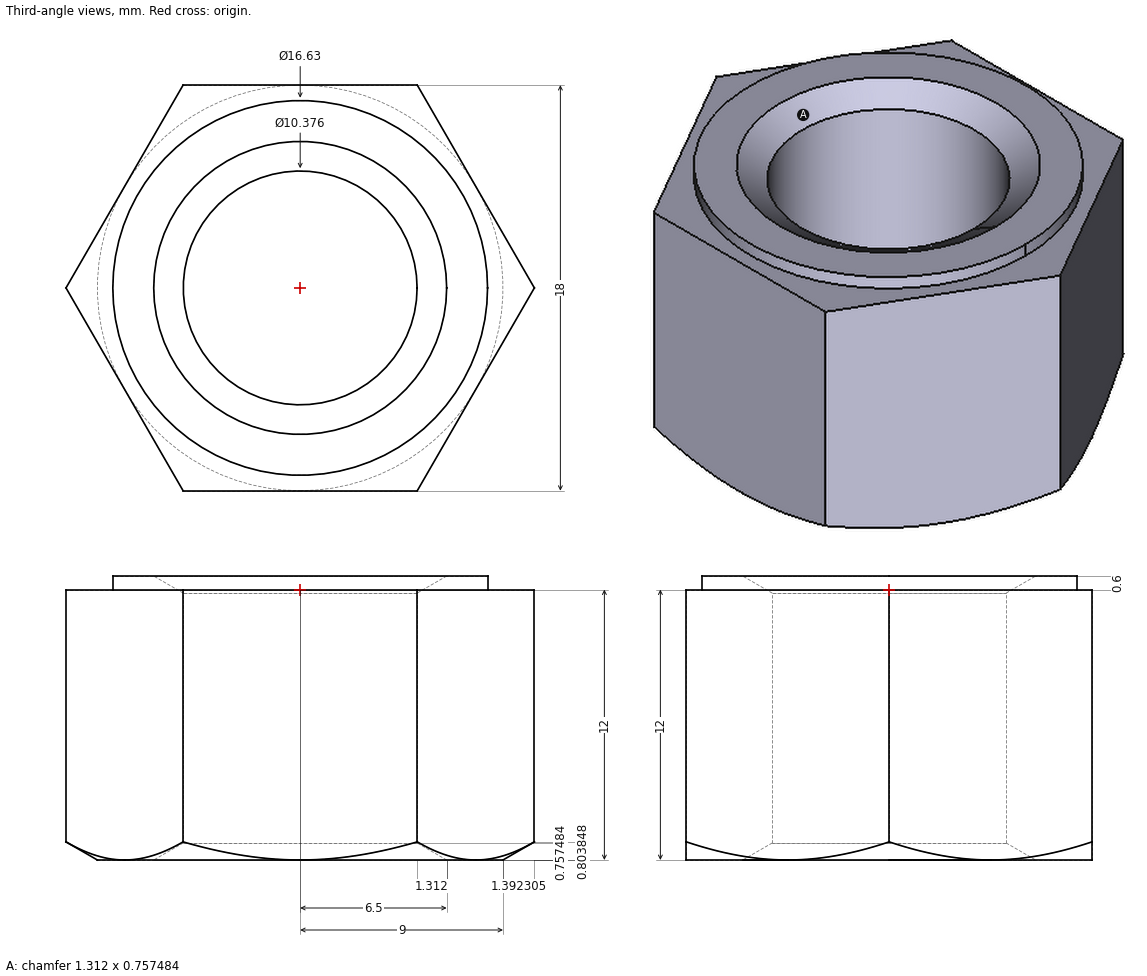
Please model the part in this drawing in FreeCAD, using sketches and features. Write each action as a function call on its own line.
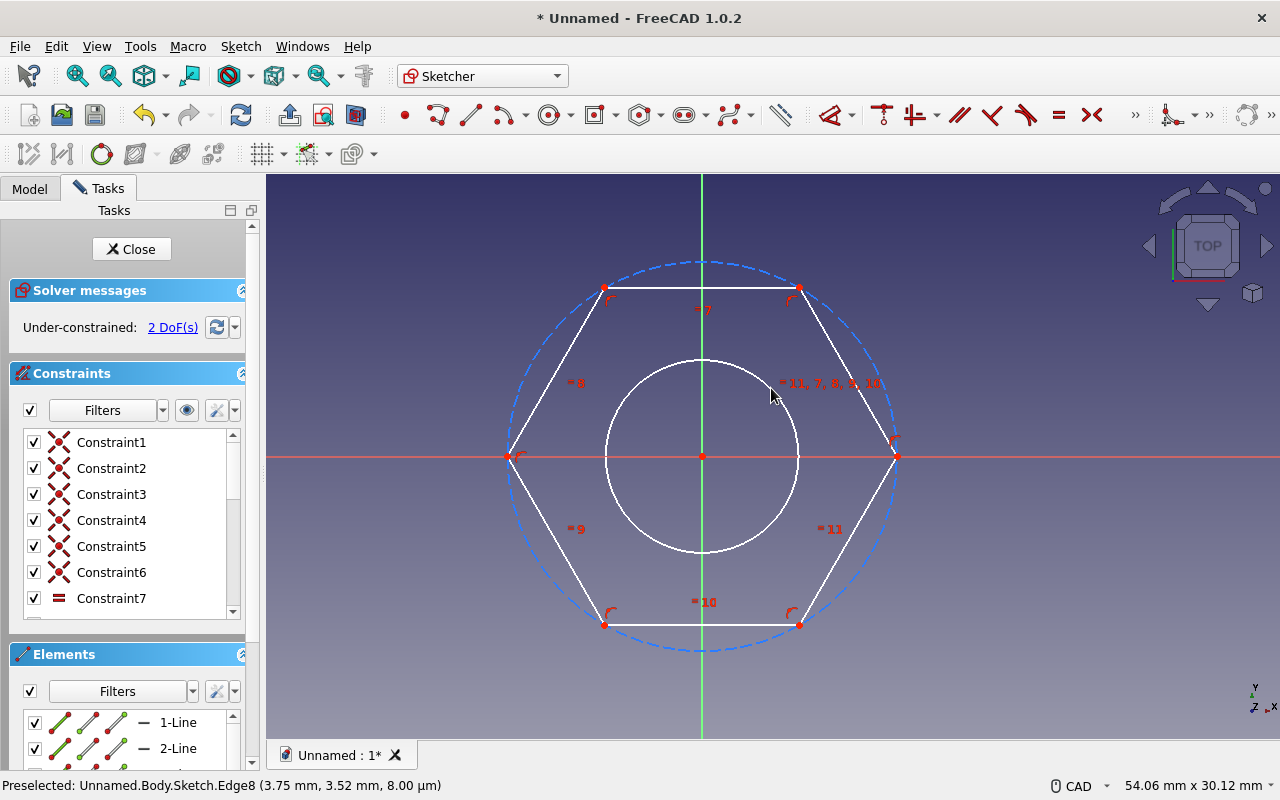
key(d)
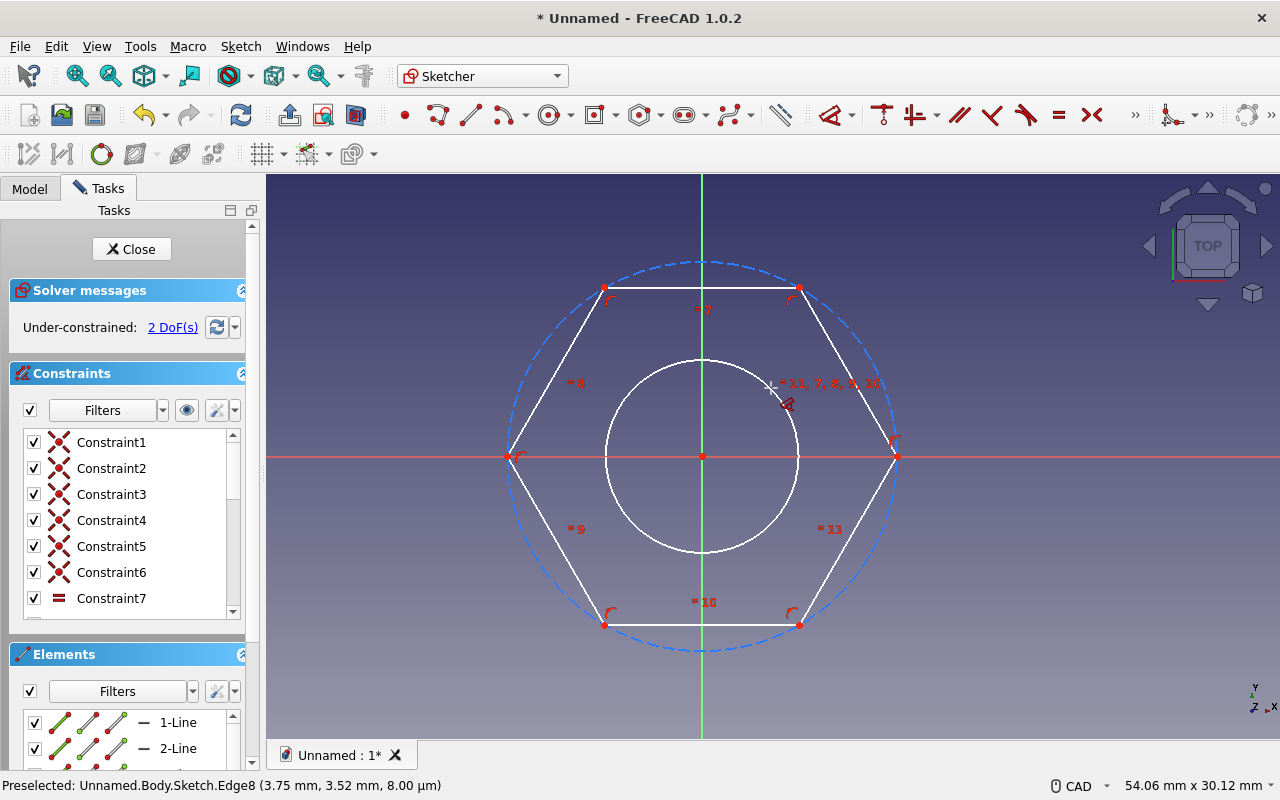
click(770, 388)
click(793, 365)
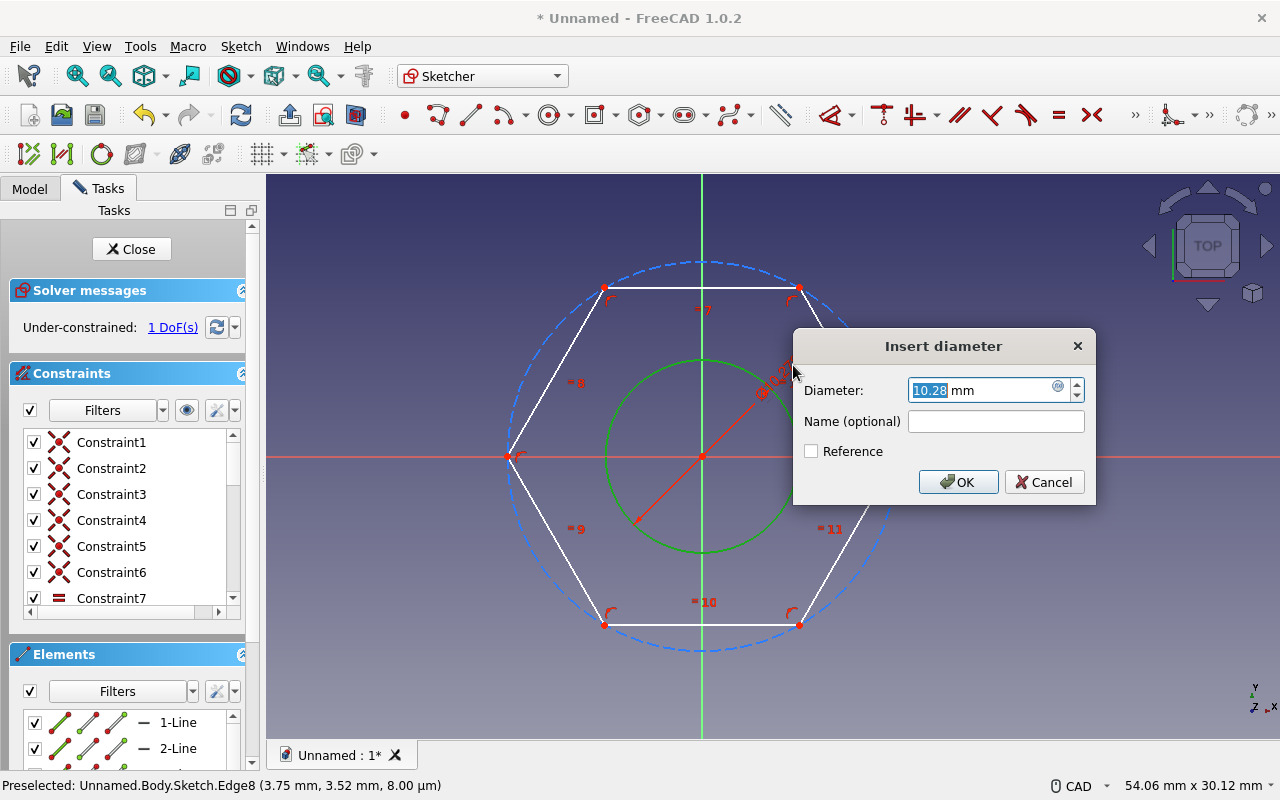
text(10.376)
key(Return)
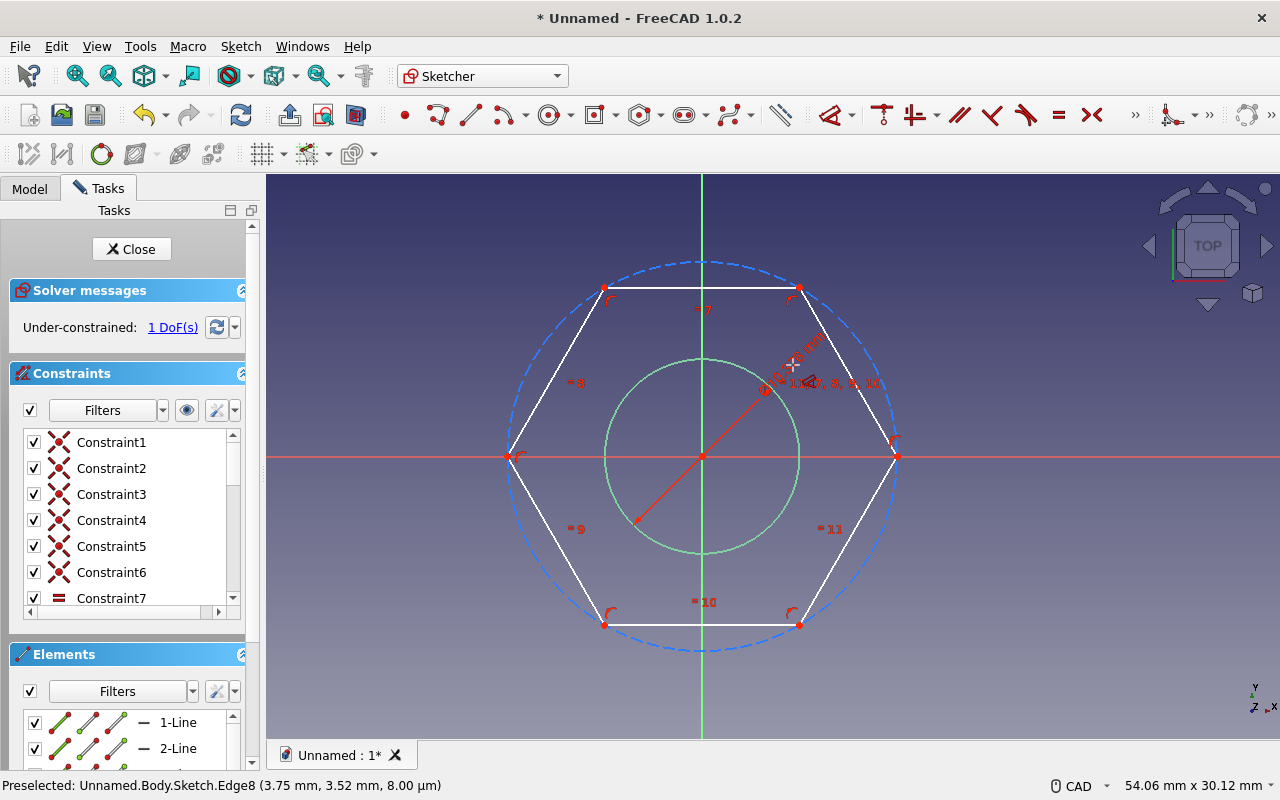
click(605, 625)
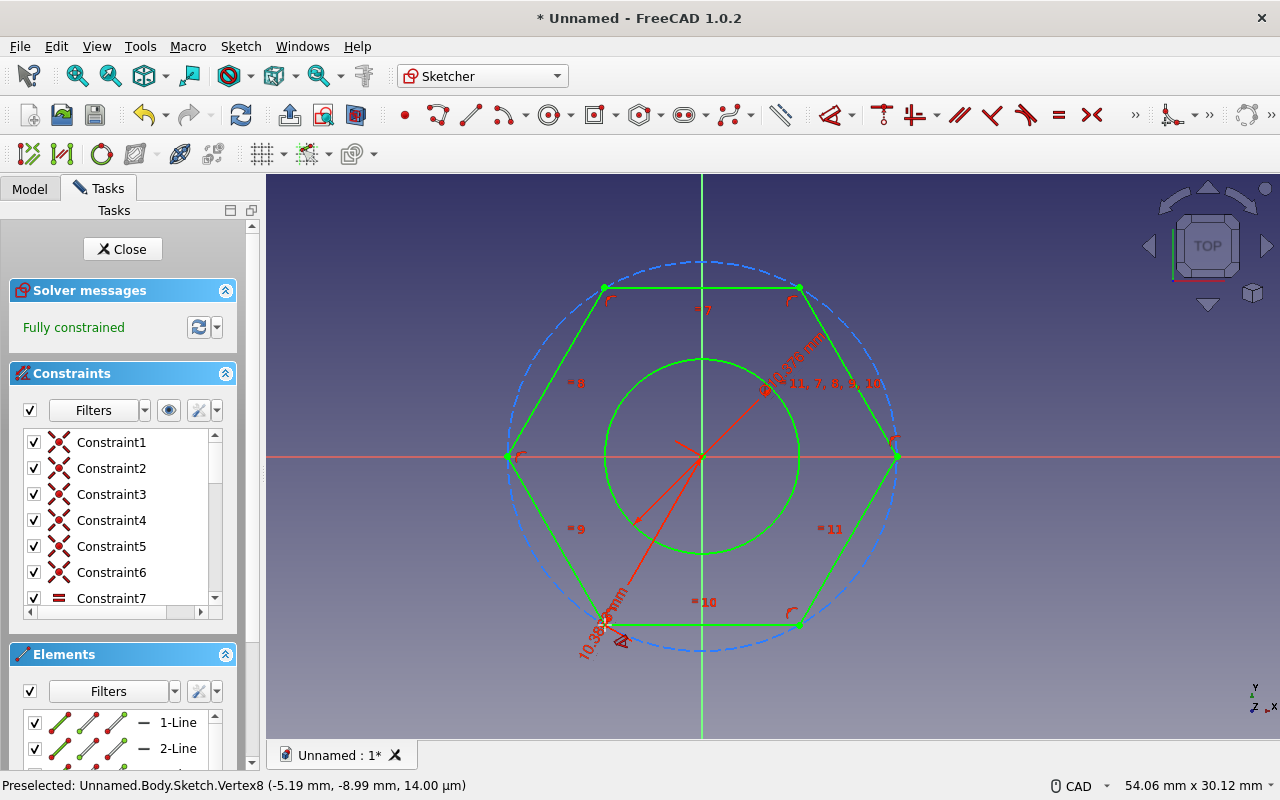
click(800, 288)
click(834, 534)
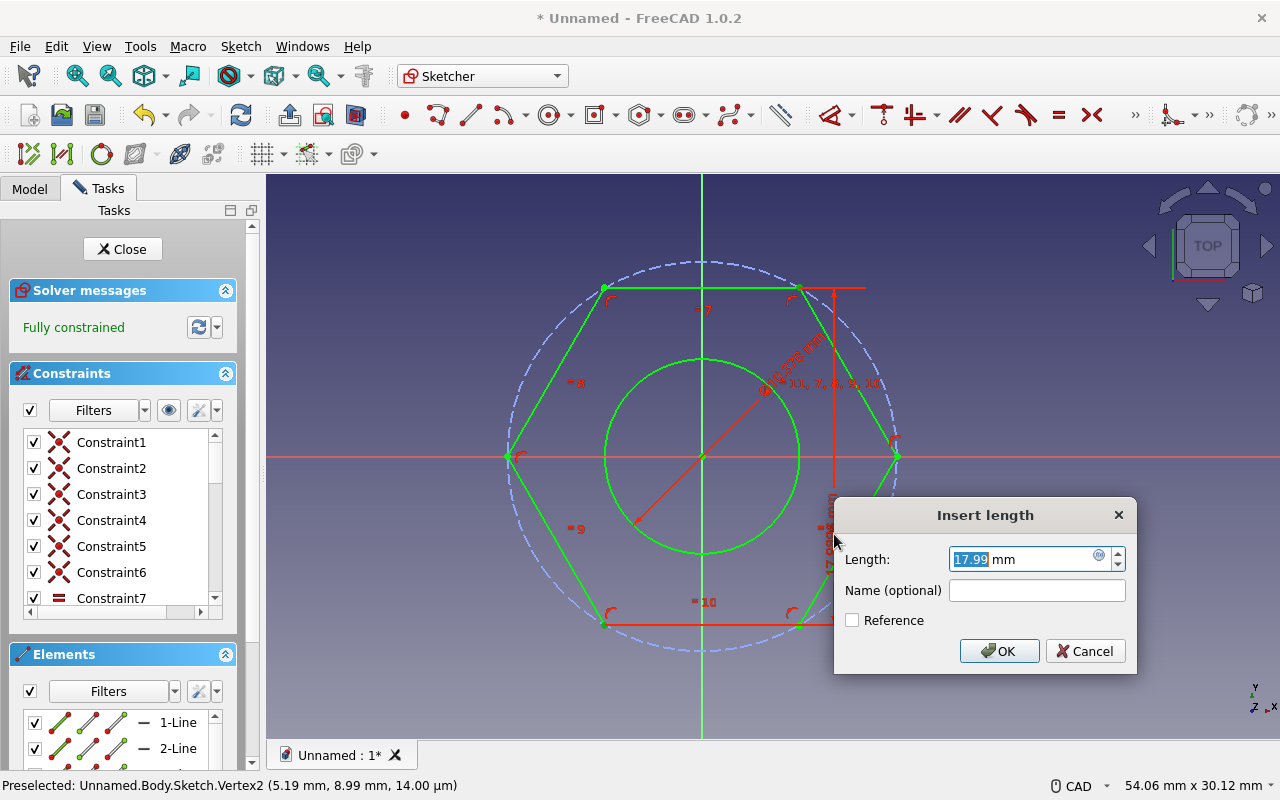
text(18)
key(Return)
key(Escape)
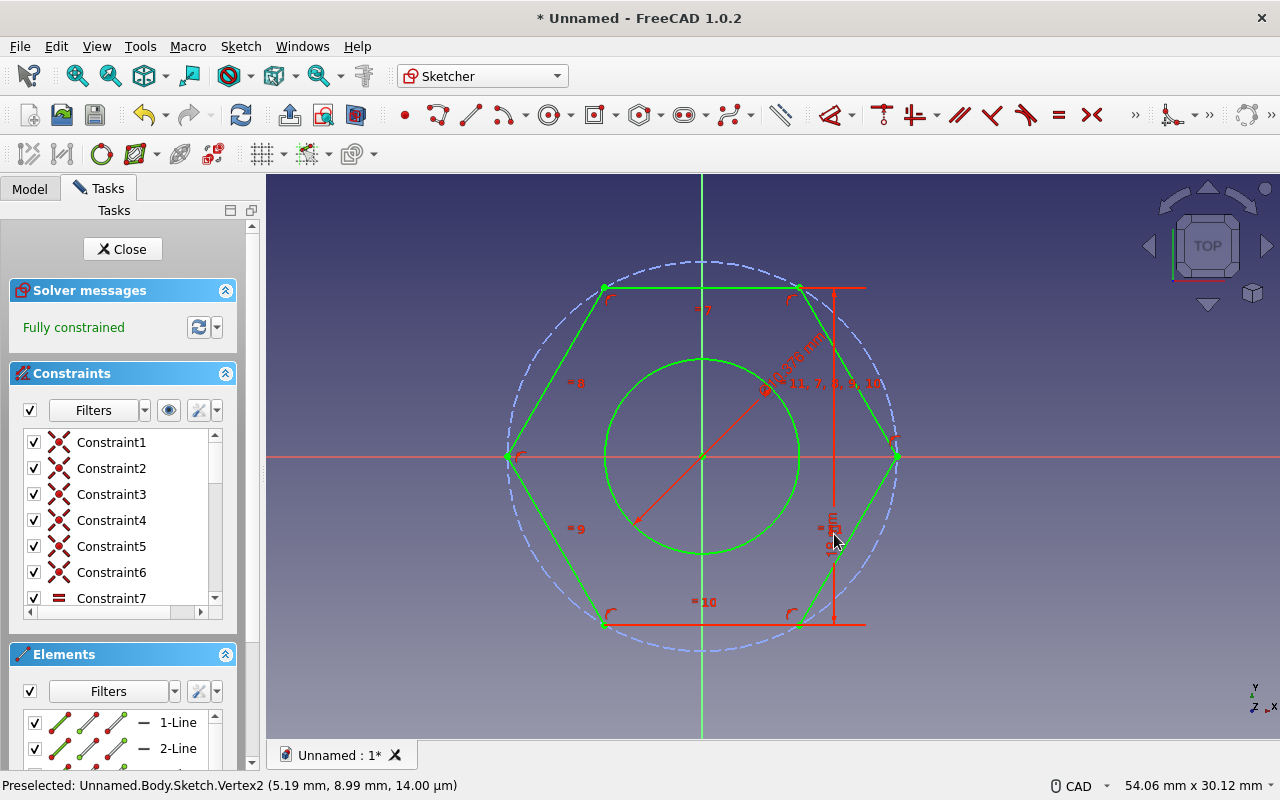
click(123, 249)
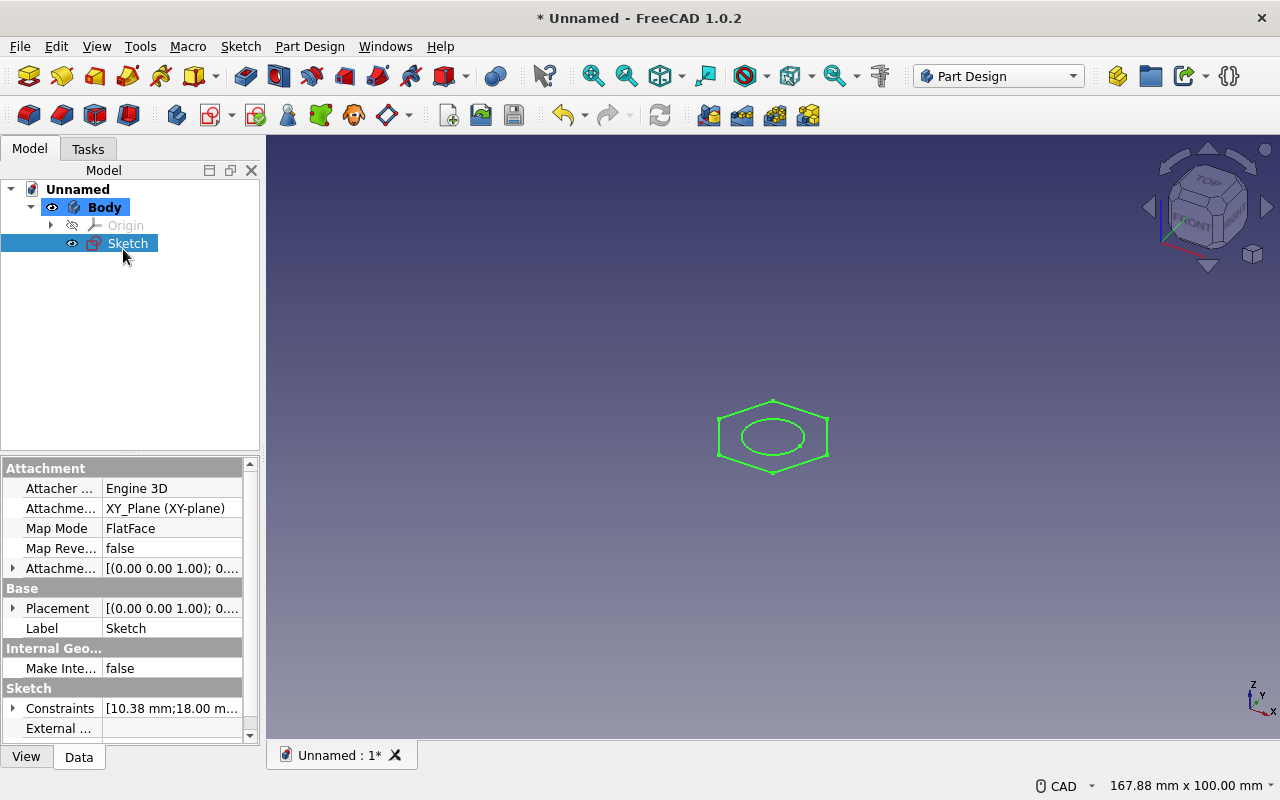
click(29, 76)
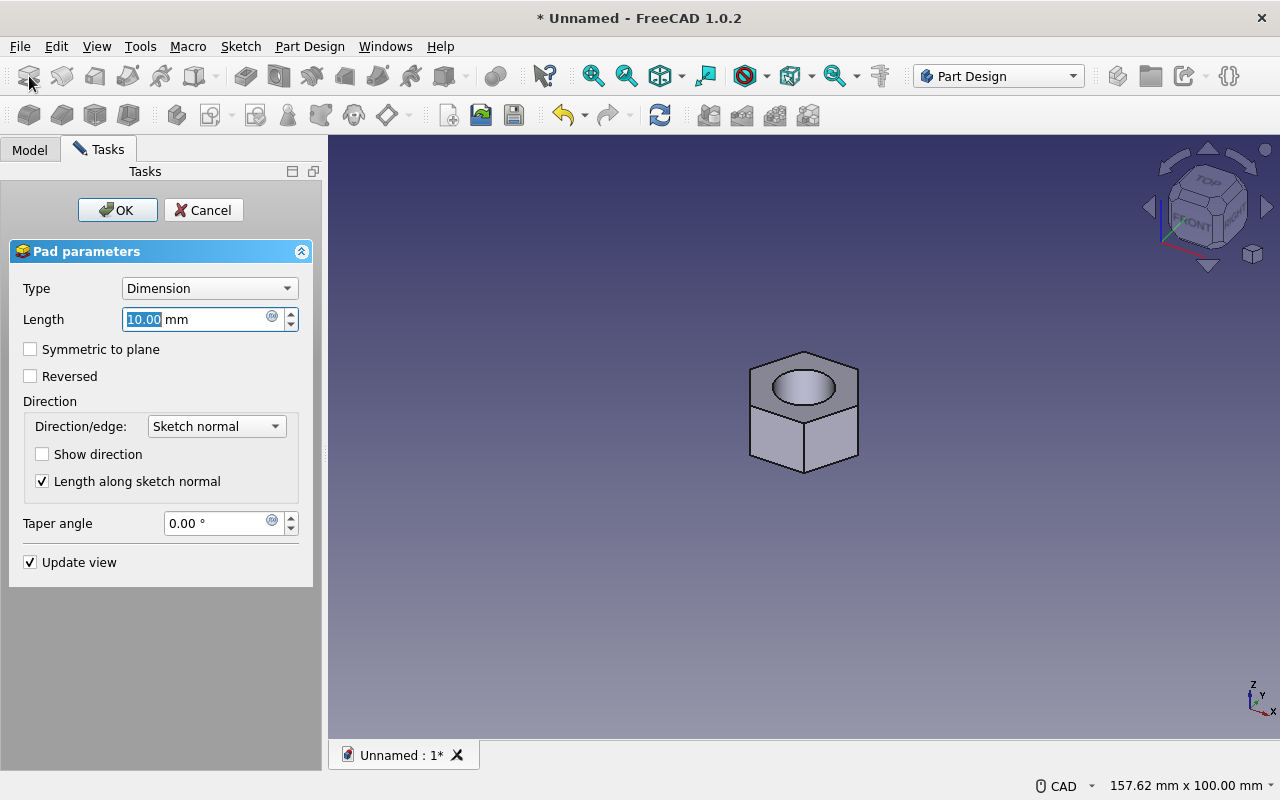
text(12)
key(Tab)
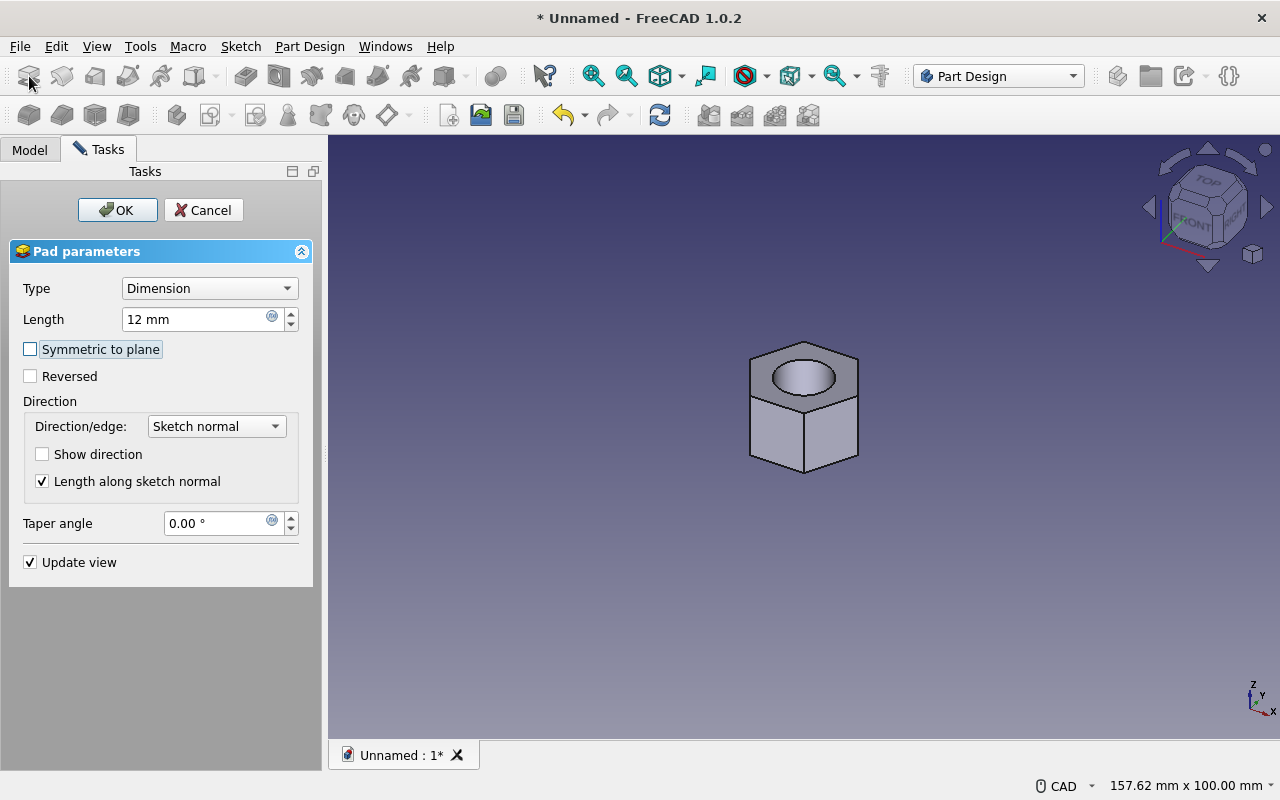
click(31, 376)